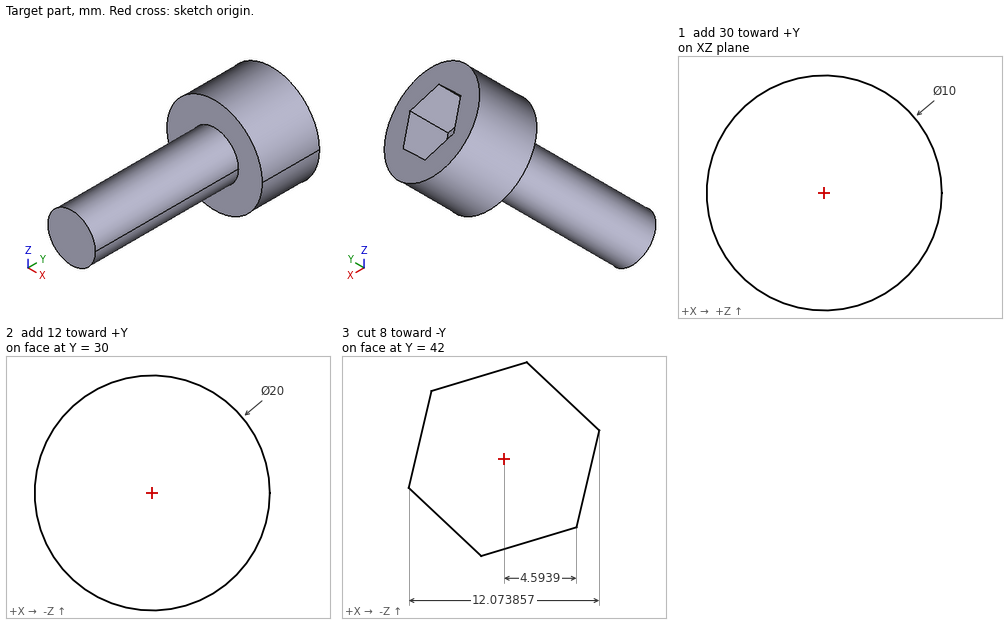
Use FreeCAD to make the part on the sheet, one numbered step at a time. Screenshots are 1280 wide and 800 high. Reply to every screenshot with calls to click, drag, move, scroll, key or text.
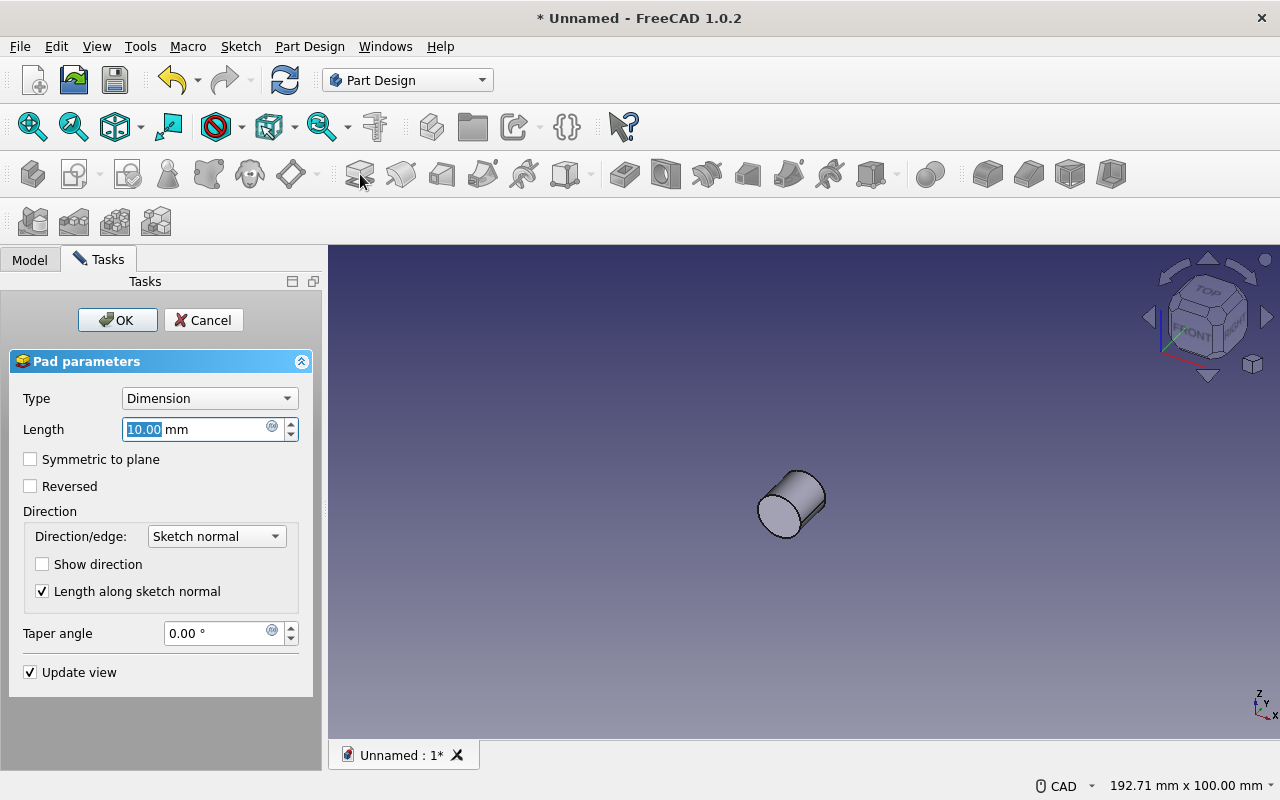
text(30)
key(Tab)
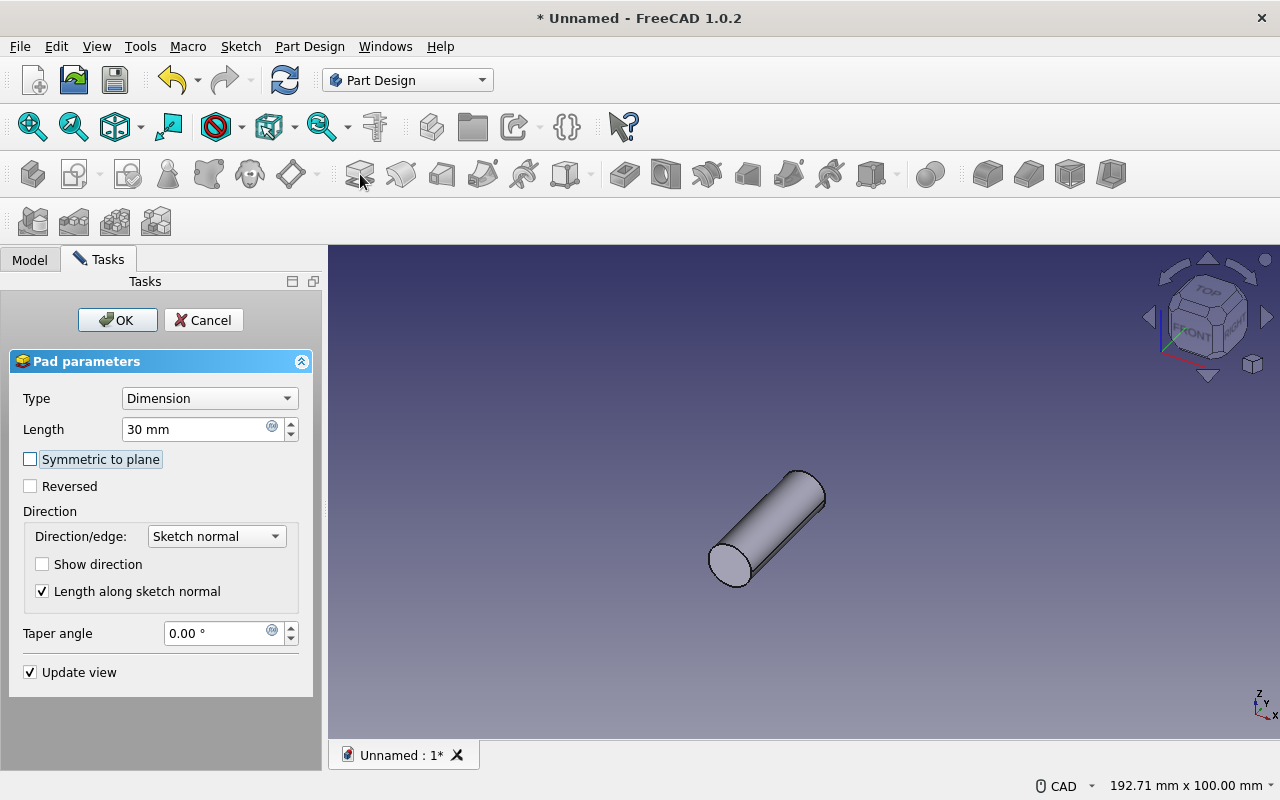
click(31, 486)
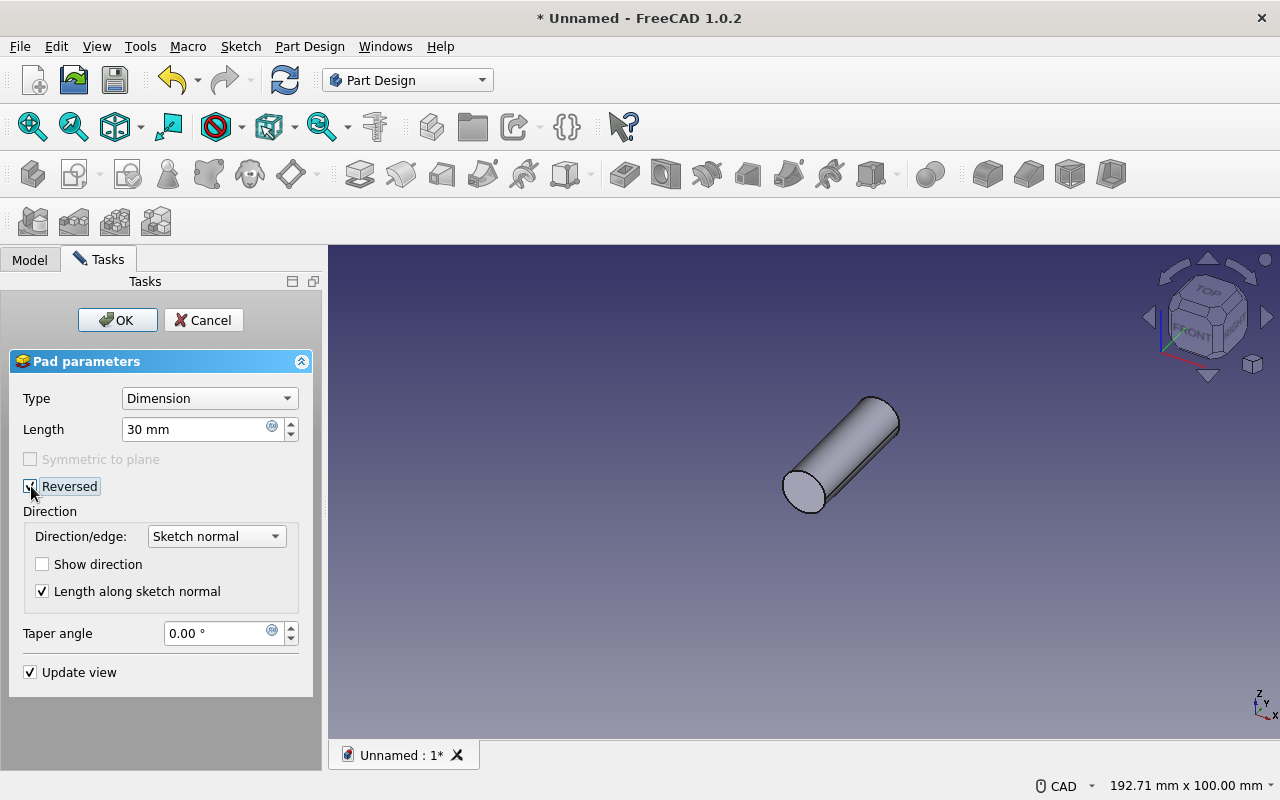
click(118, 320)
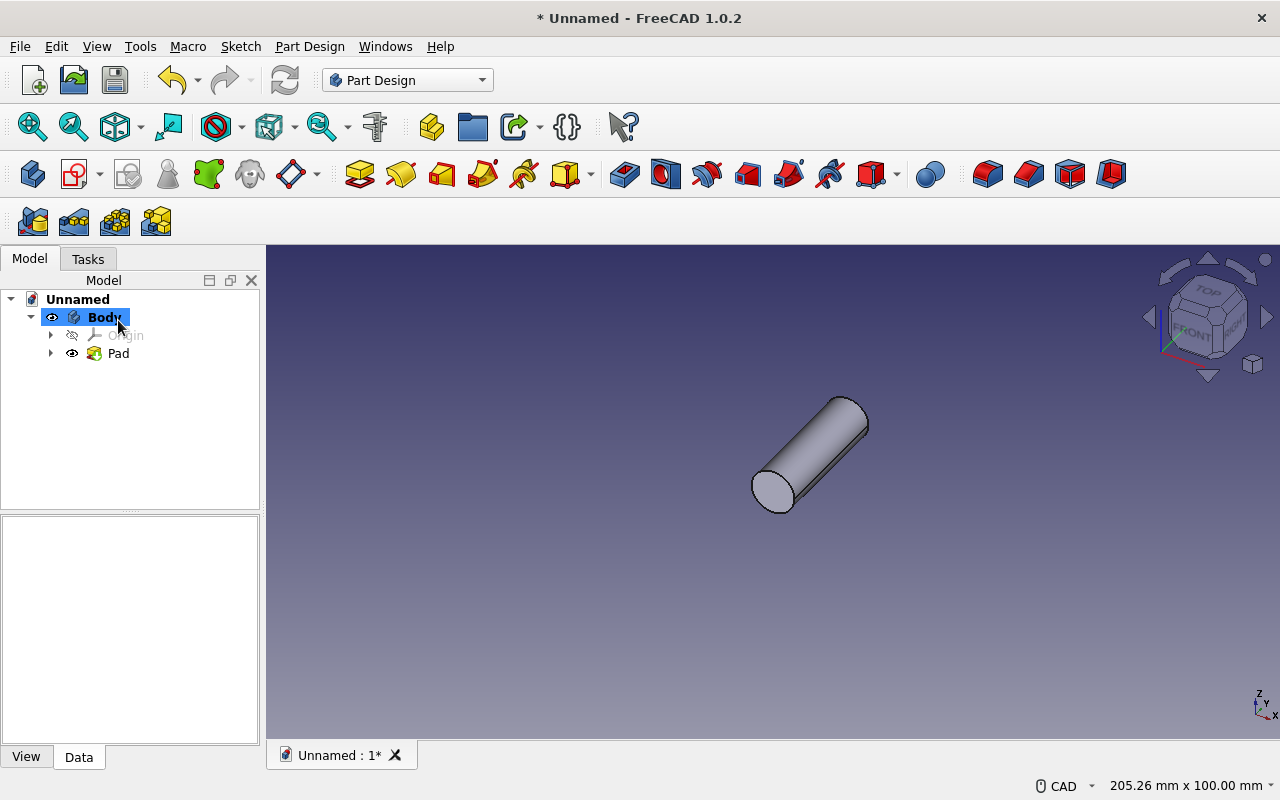
click(33, 128)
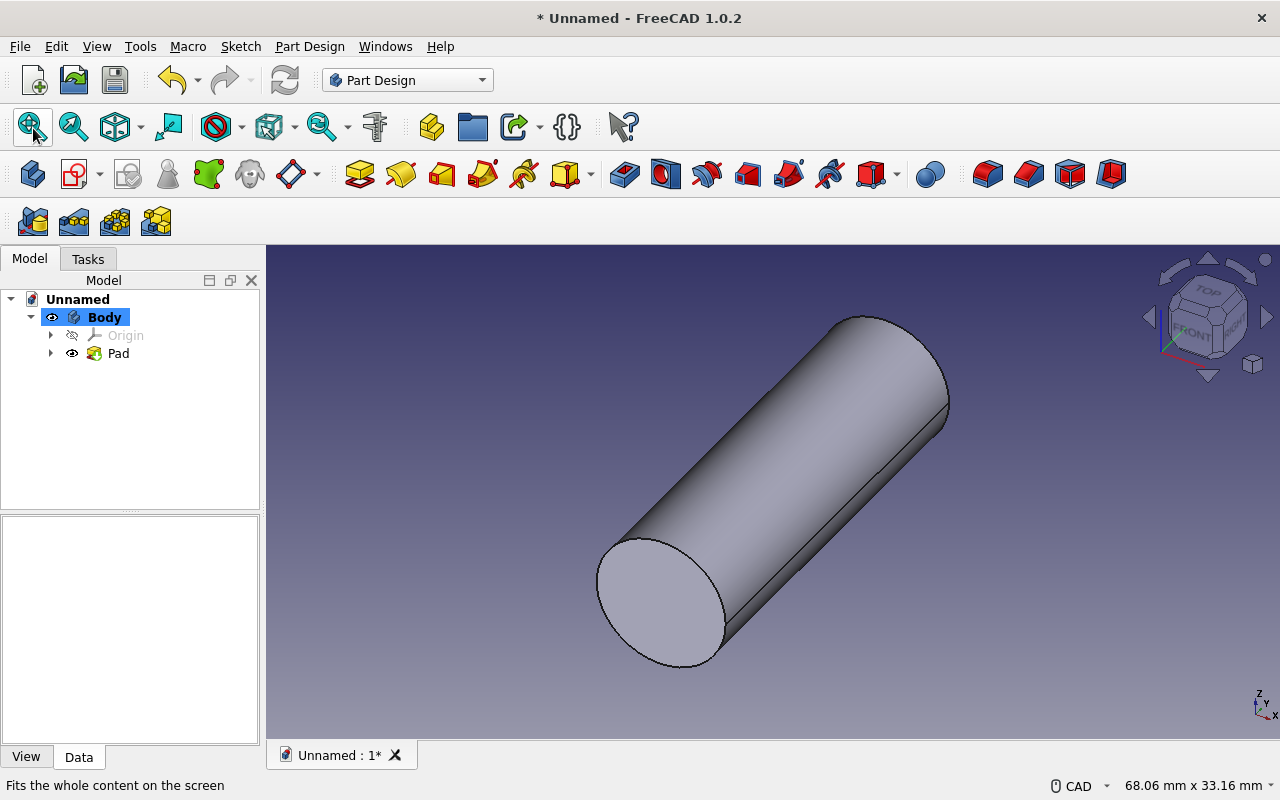
key(4)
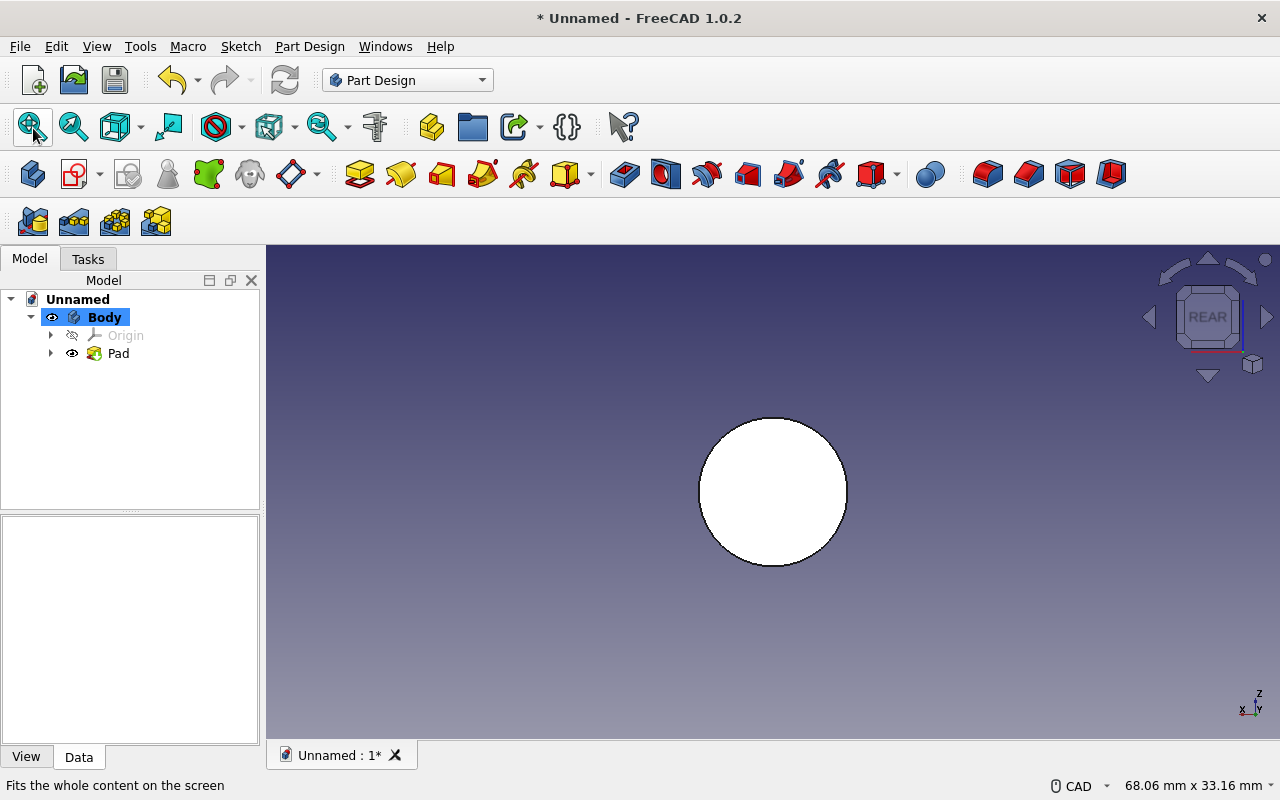
click(33, 128)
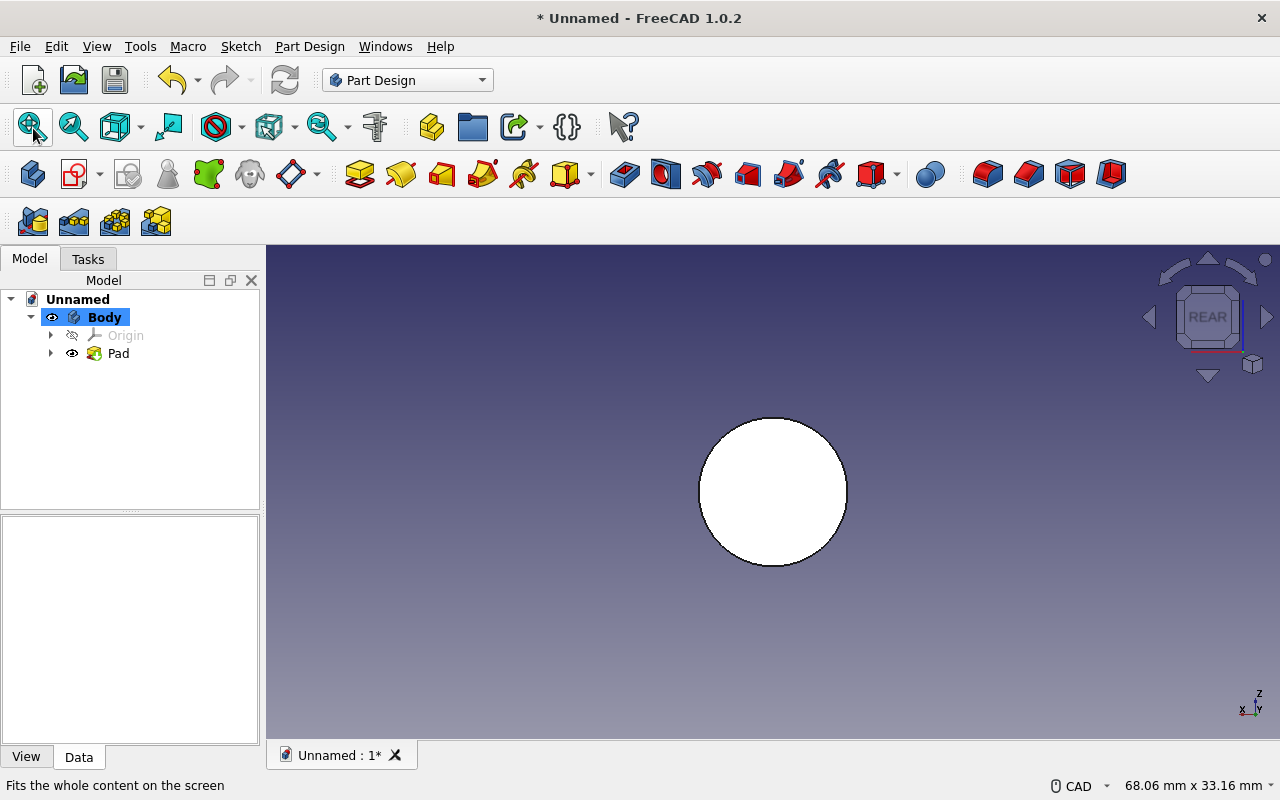
click(773, 491)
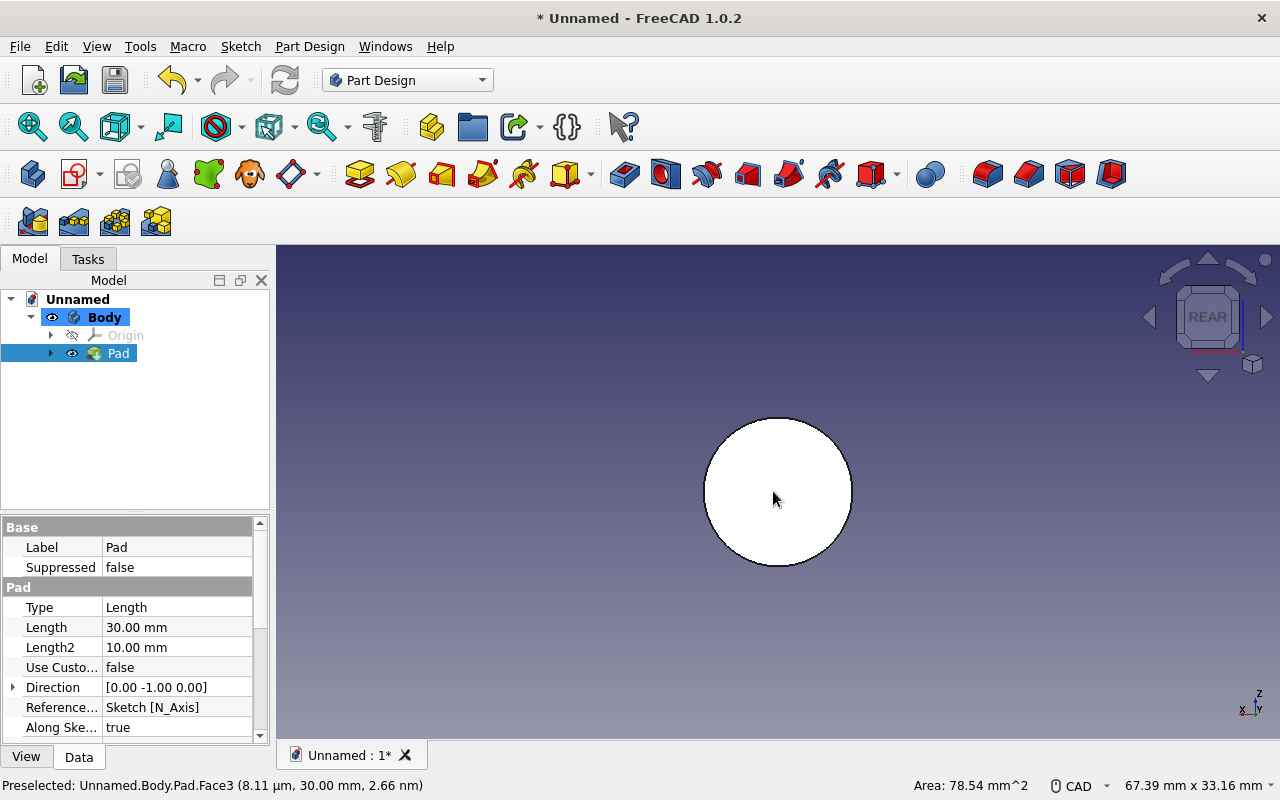
click(74, 174)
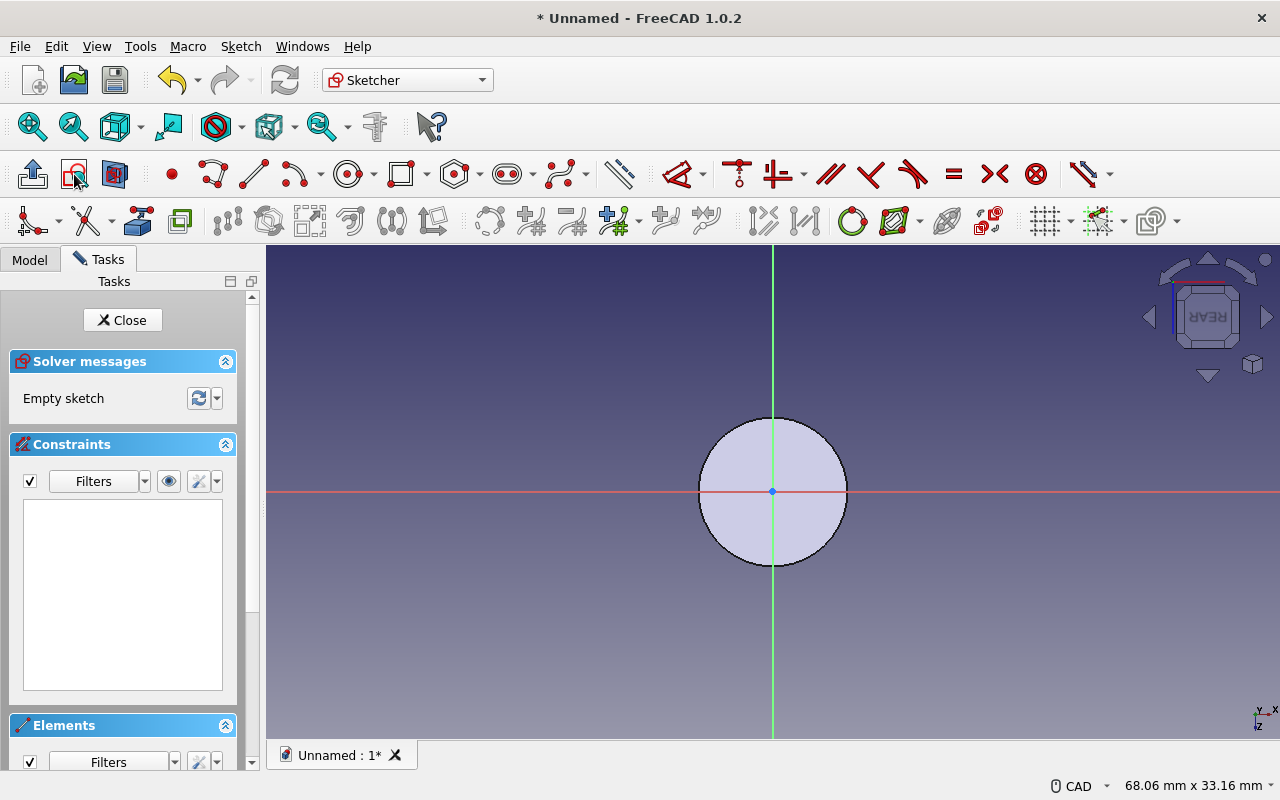
click(348, 174)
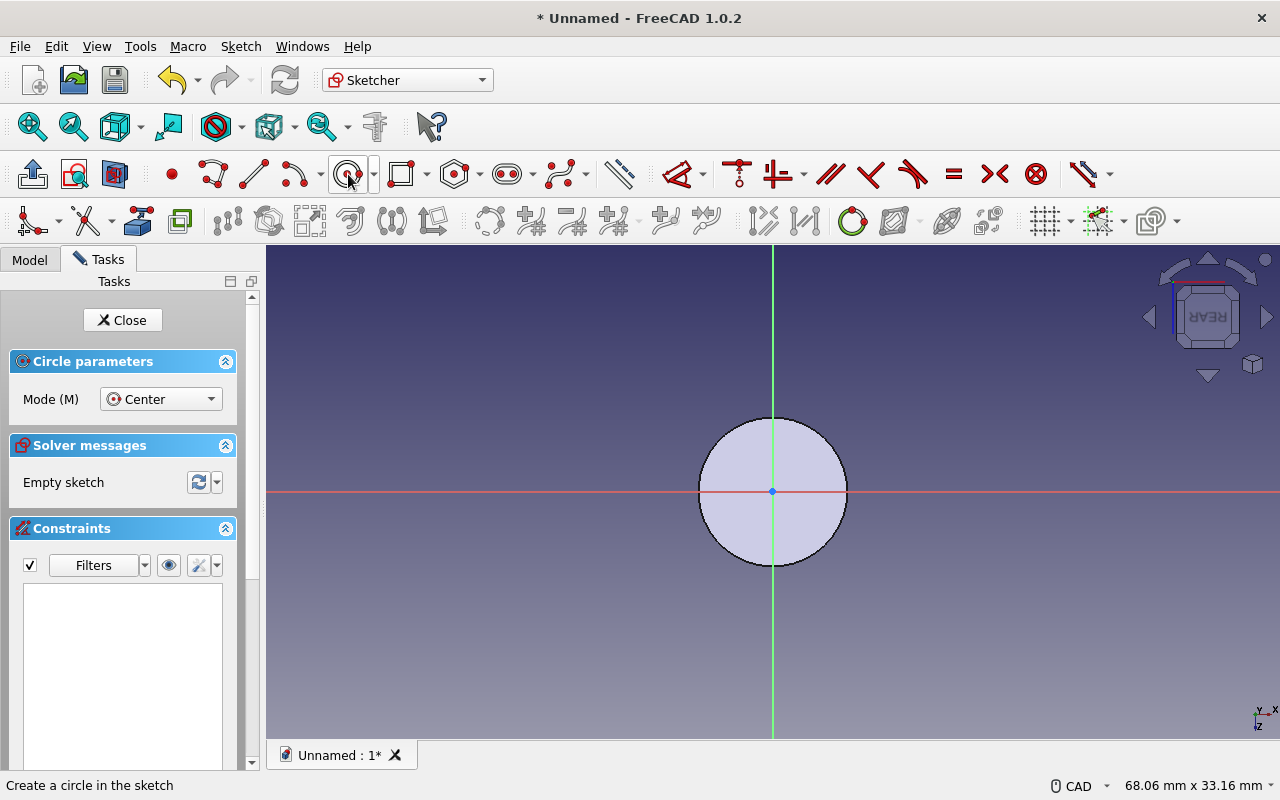
click(773, 492)
move(878, 387)